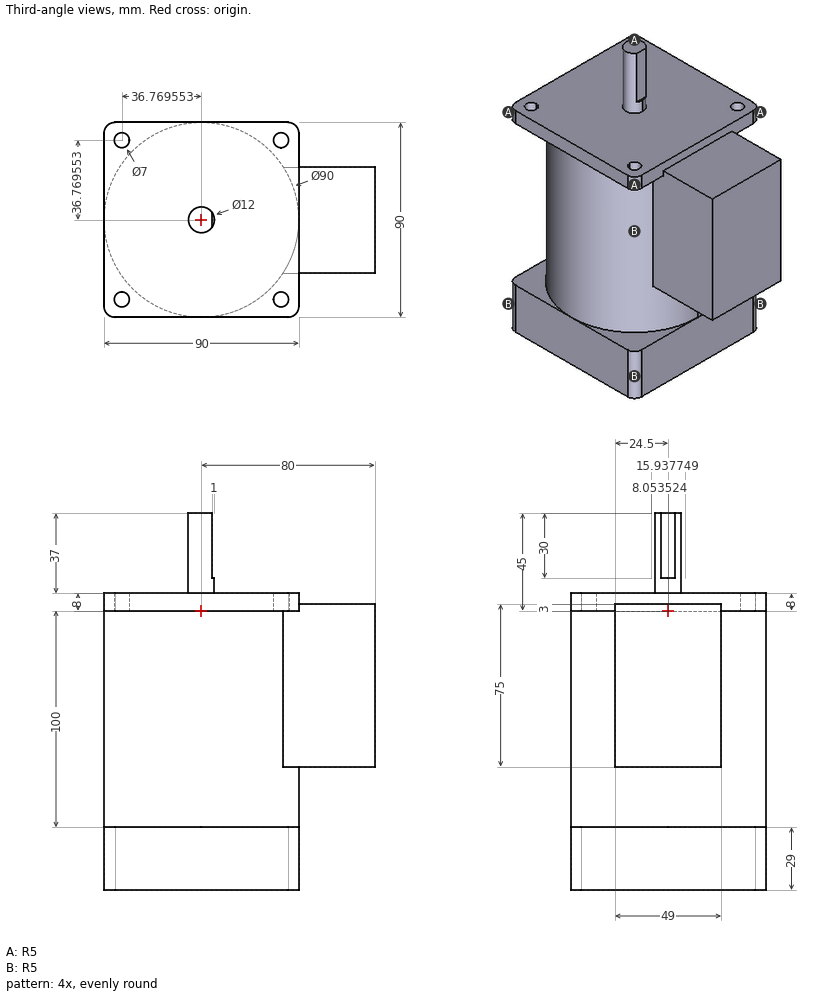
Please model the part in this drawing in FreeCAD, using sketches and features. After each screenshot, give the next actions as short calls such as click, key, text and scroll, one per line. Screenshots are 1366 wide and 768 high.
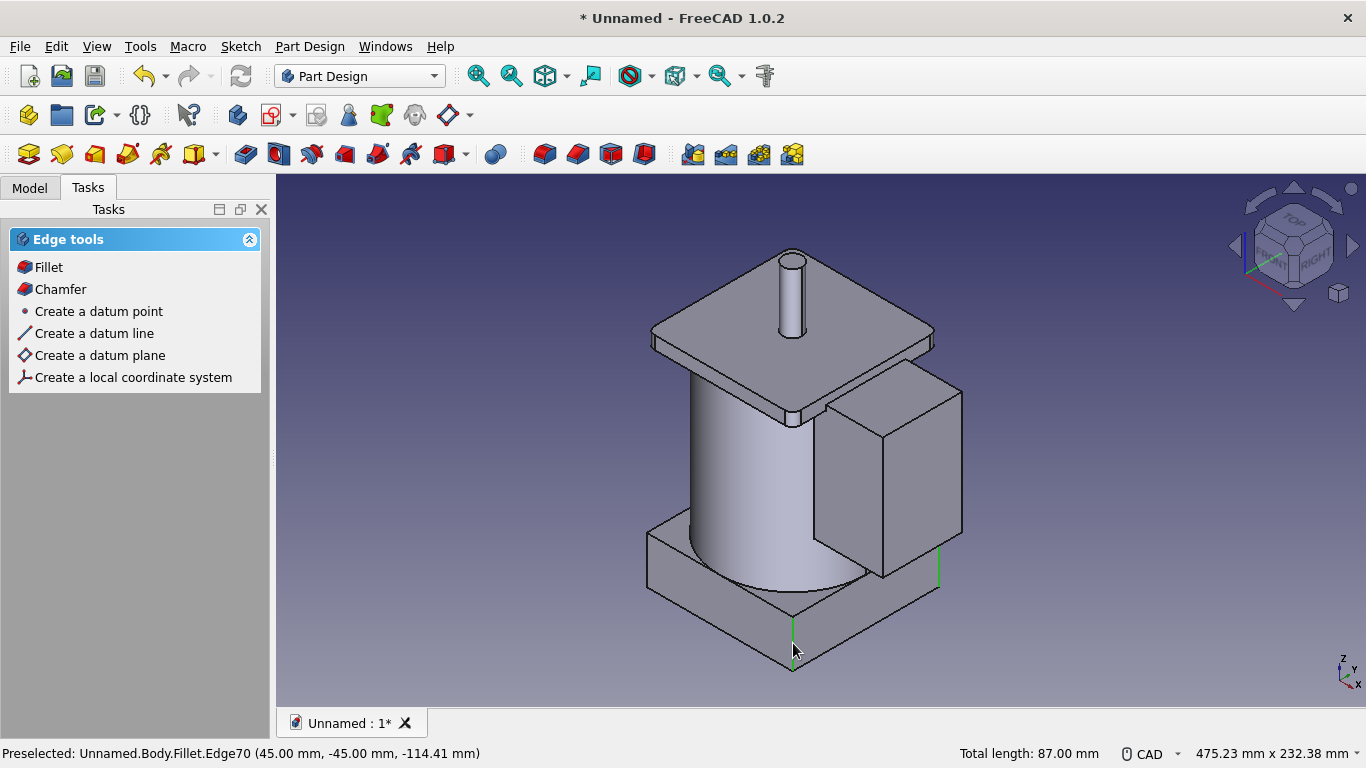
key(2)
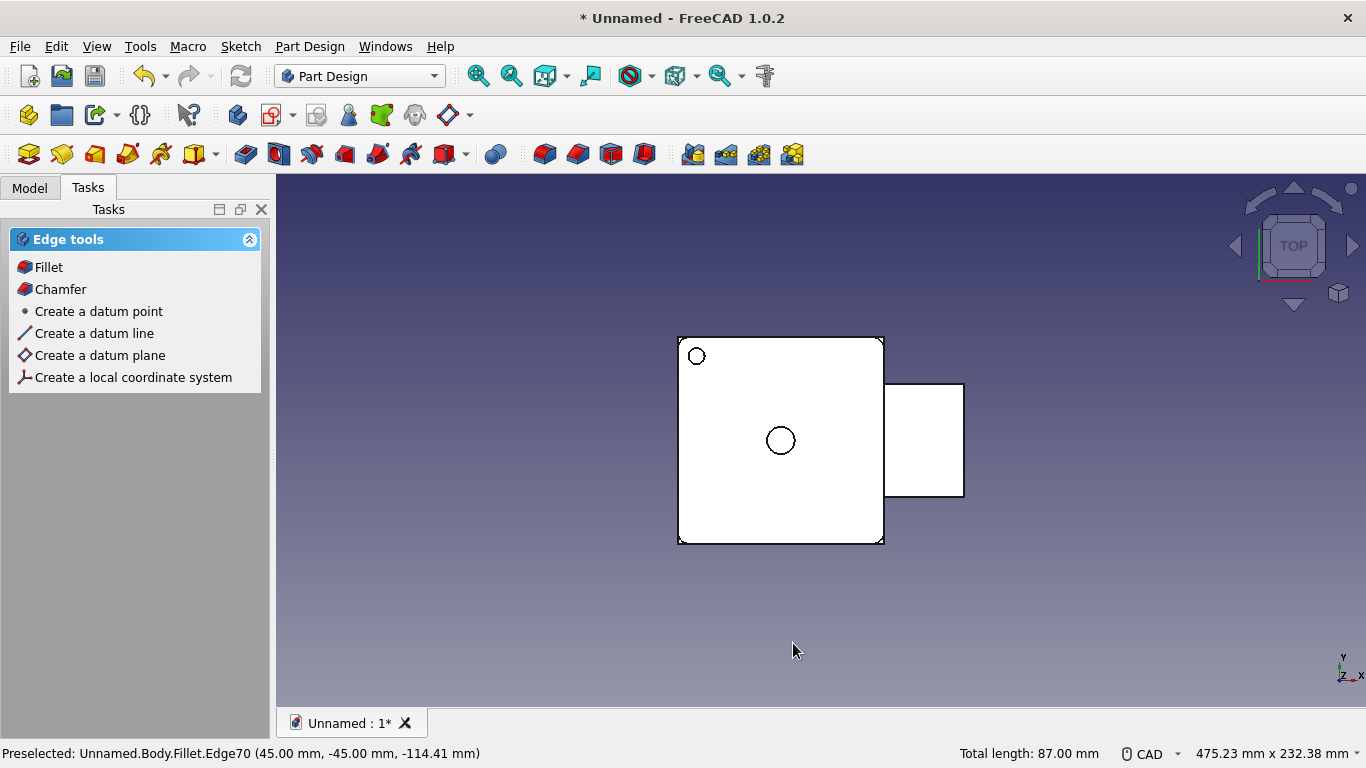
key(v)
key(f)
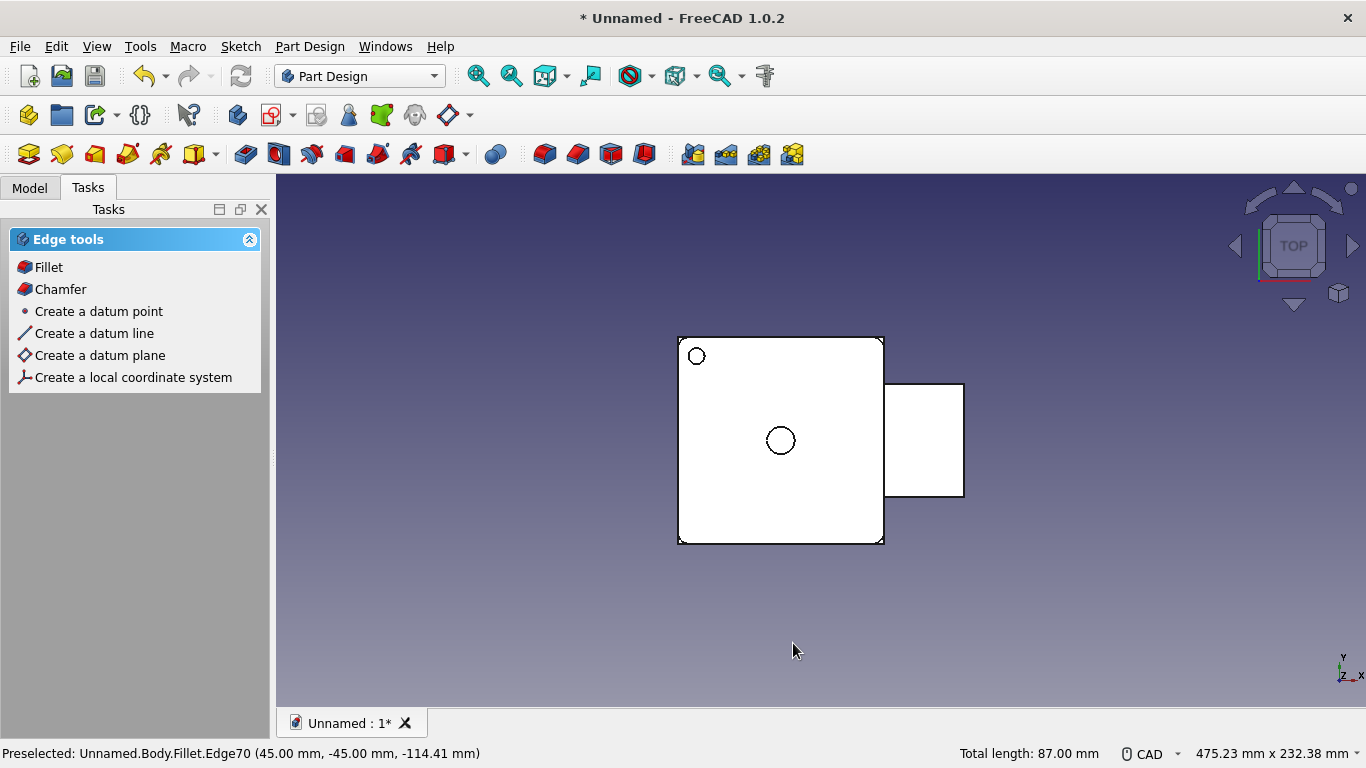
key(1)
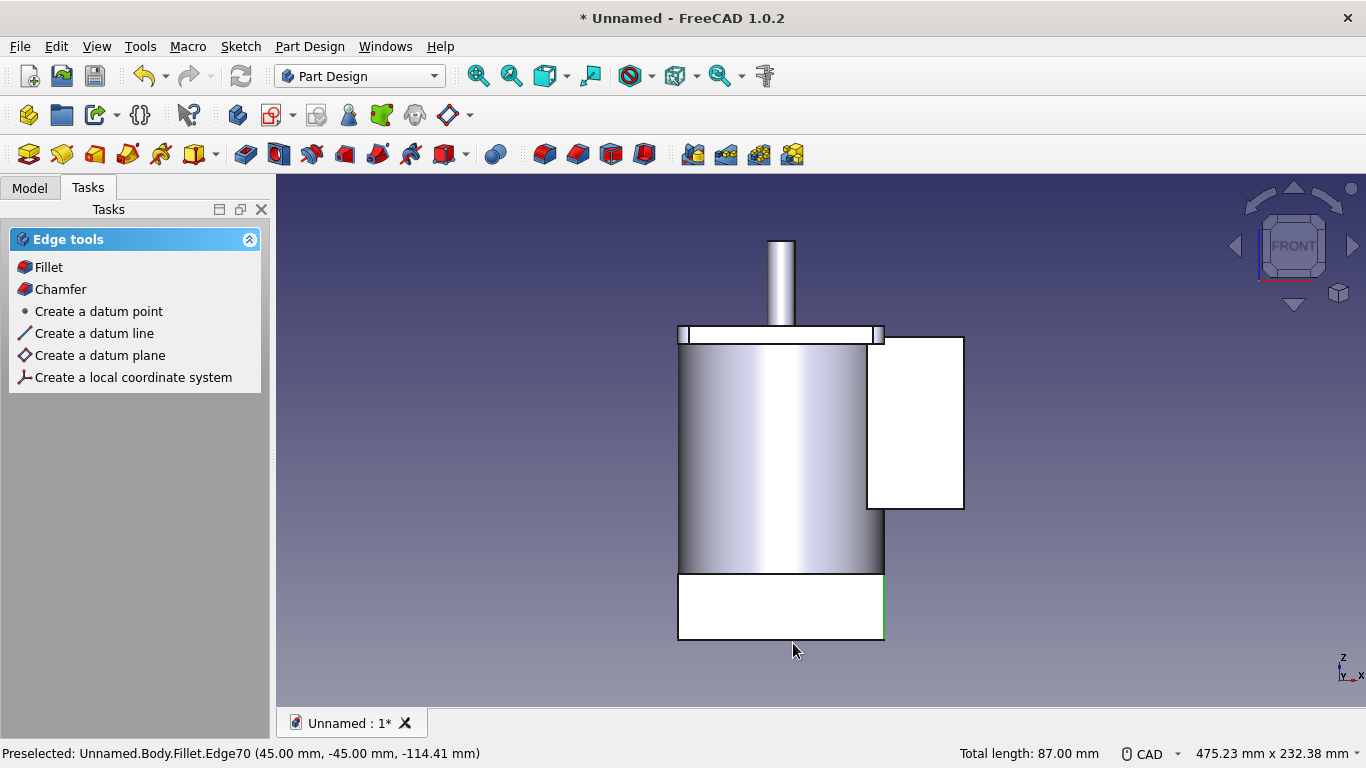
click(678, 606, ctrl)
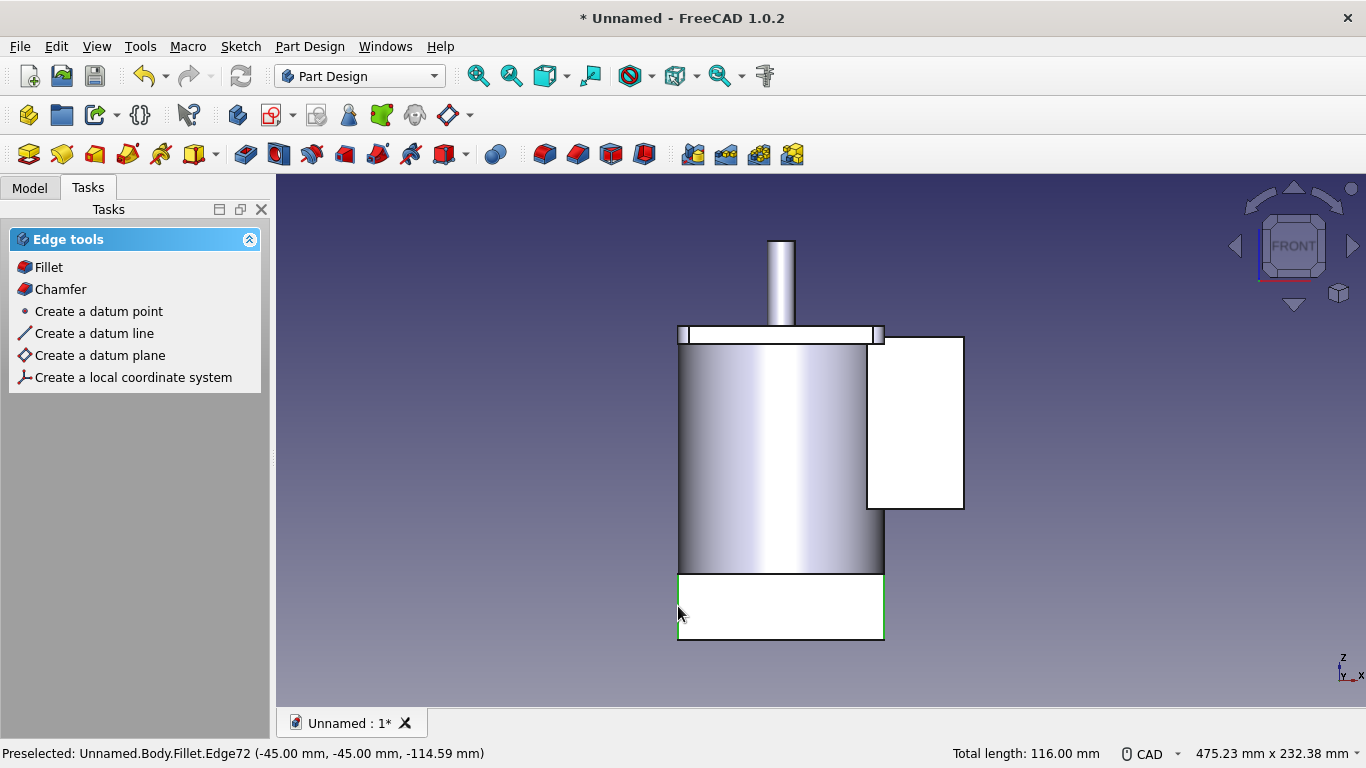
click(545, 154)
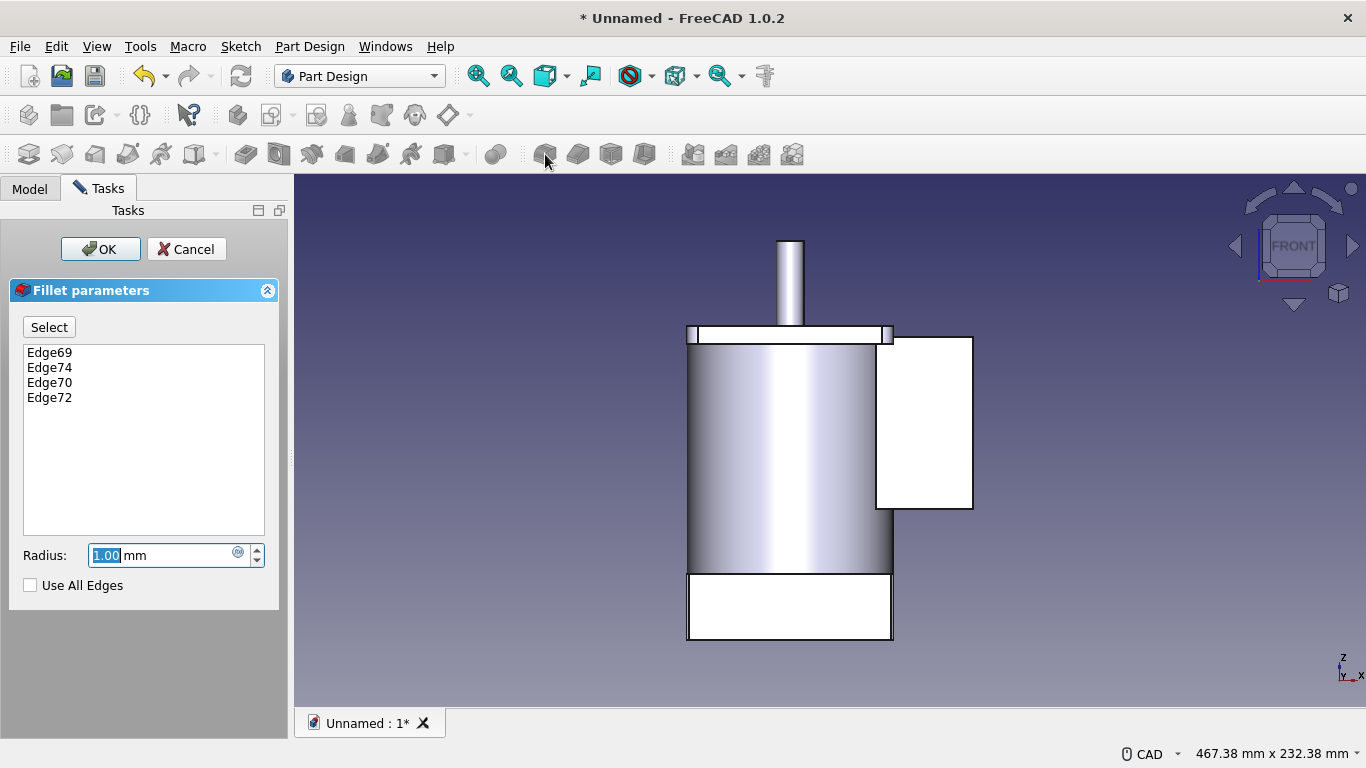
text(5)
key(Tab)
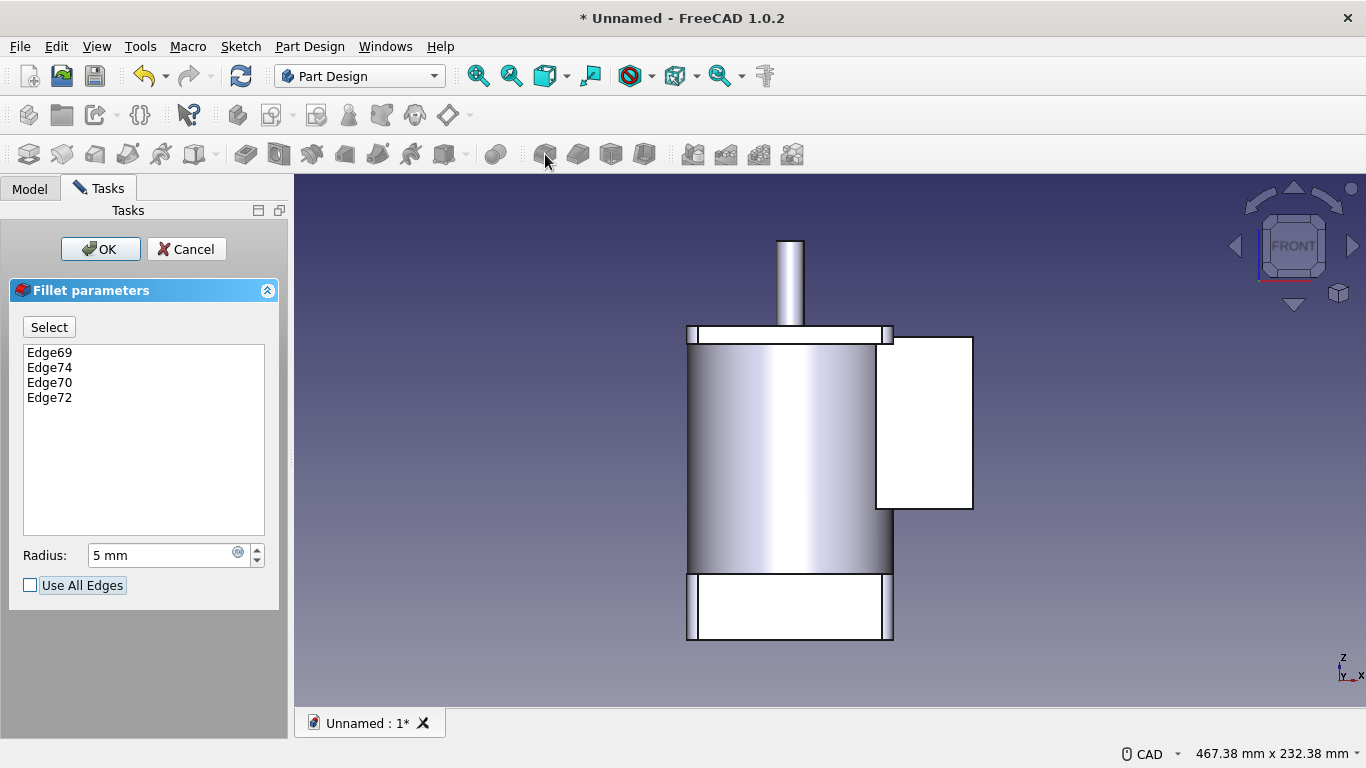
click(101, 249)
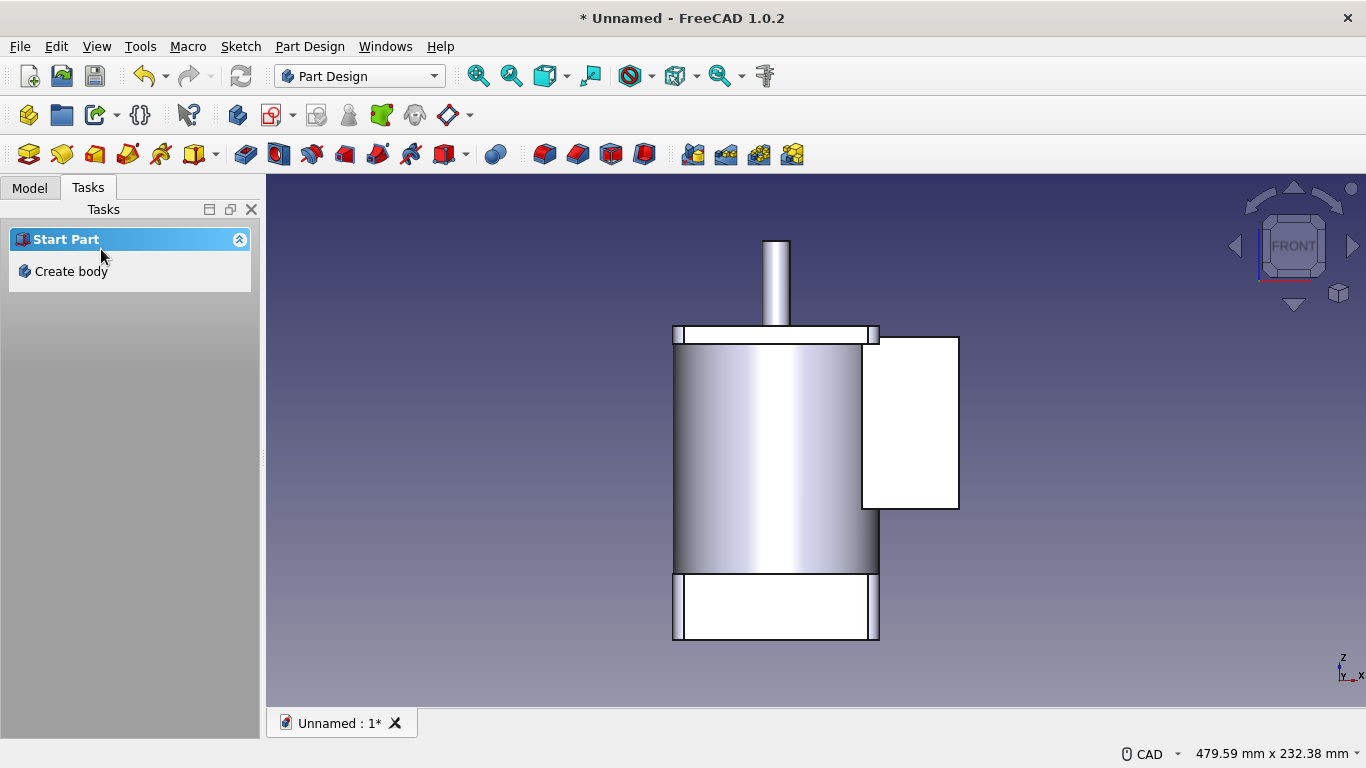
click(30, 188)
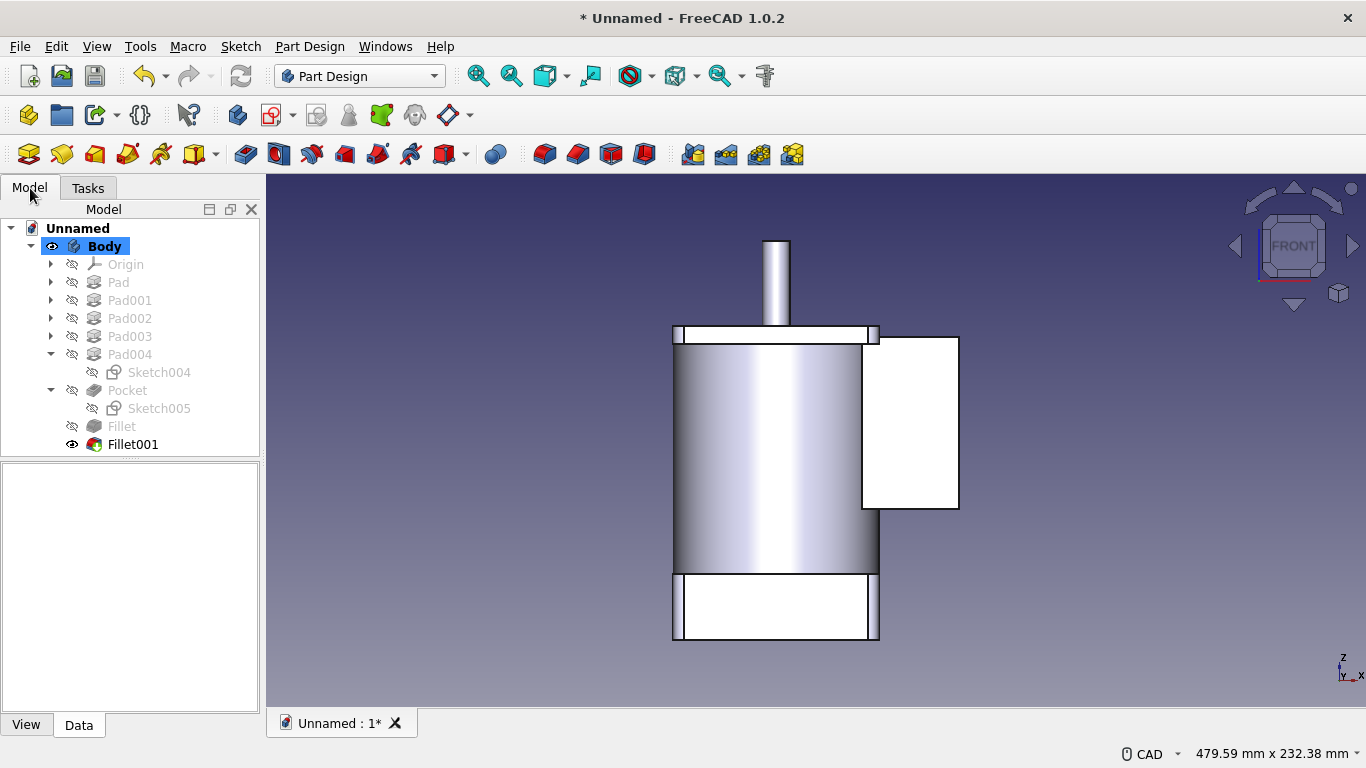
click(51, 264)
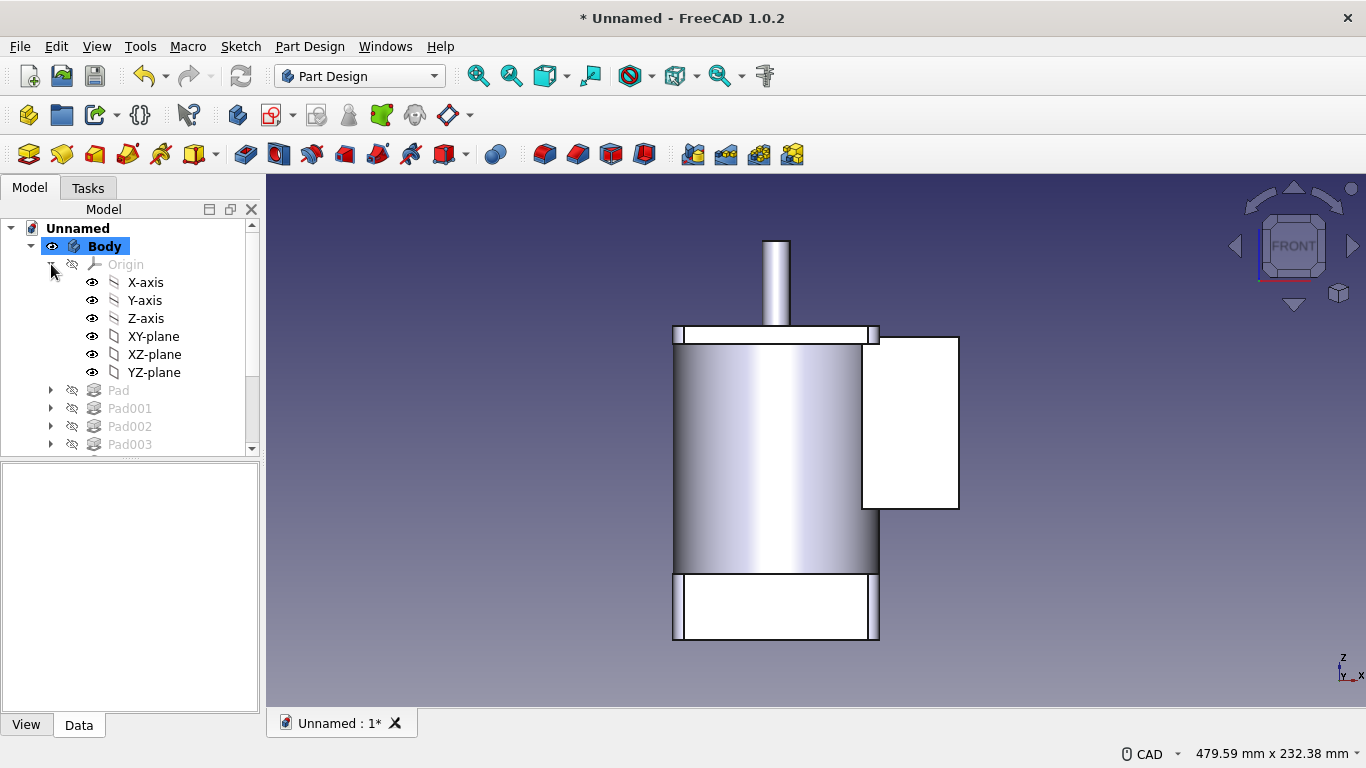
click(137, 372)